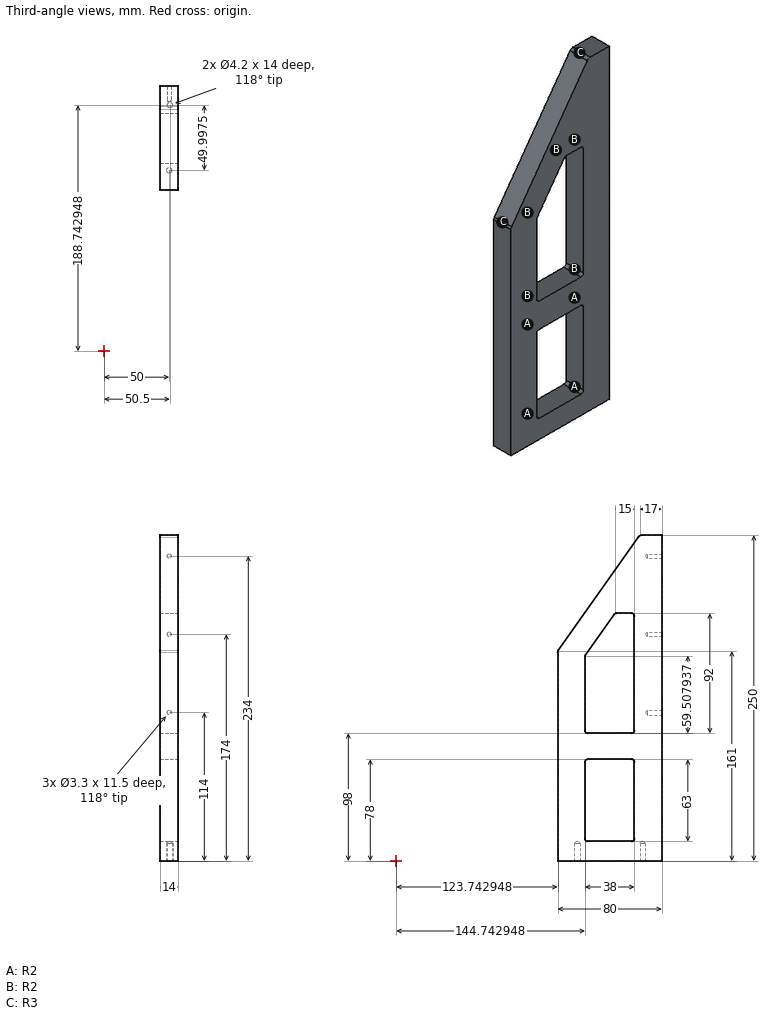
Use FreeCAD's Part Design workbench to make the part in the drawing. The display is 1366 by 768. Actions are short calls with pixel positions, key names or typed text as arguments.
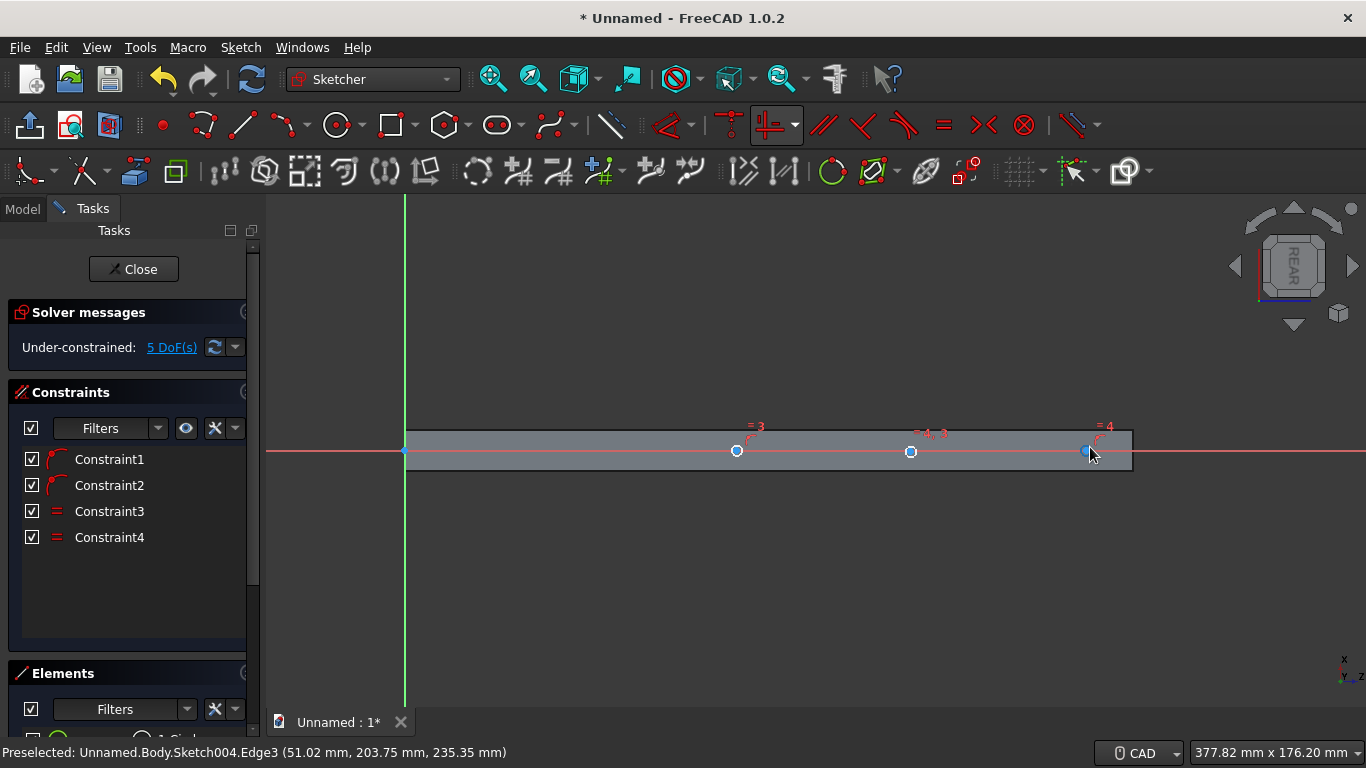
click(911, 452)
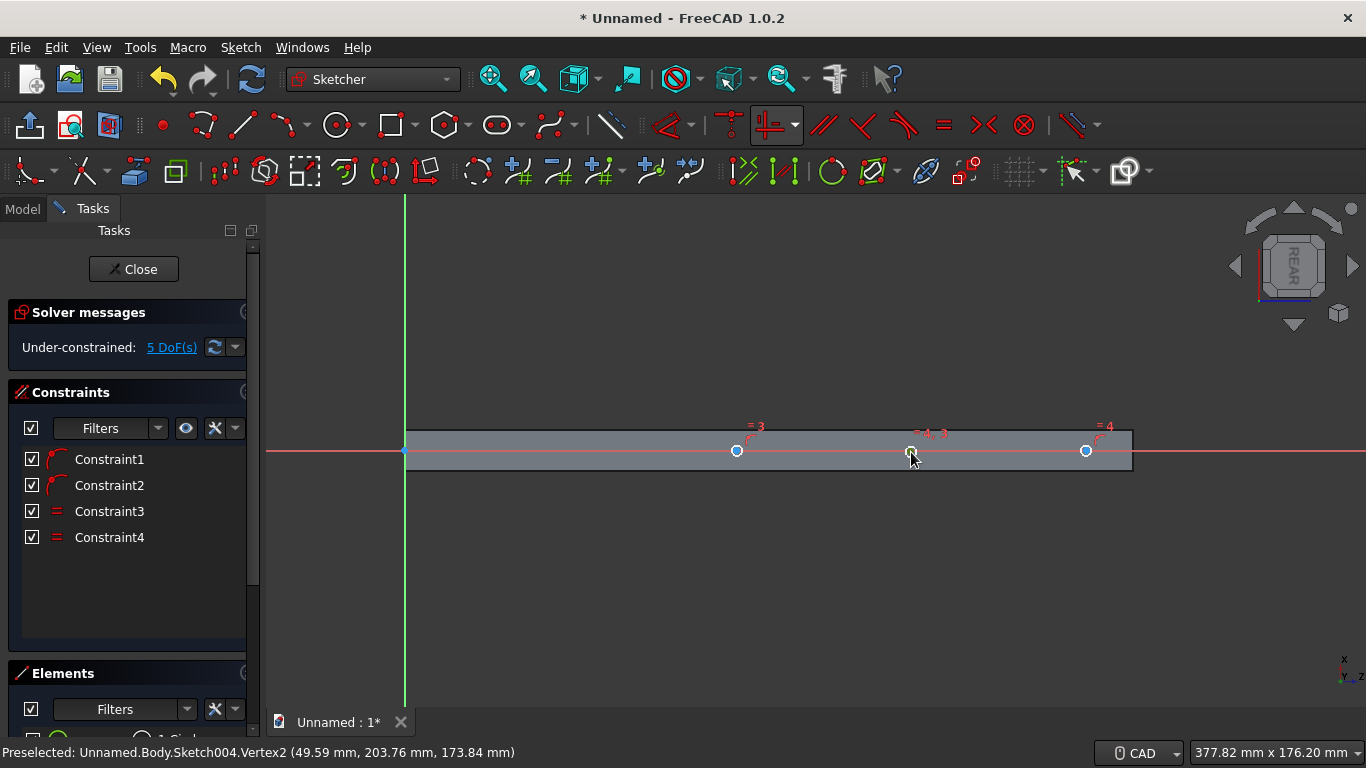
click(359, 451)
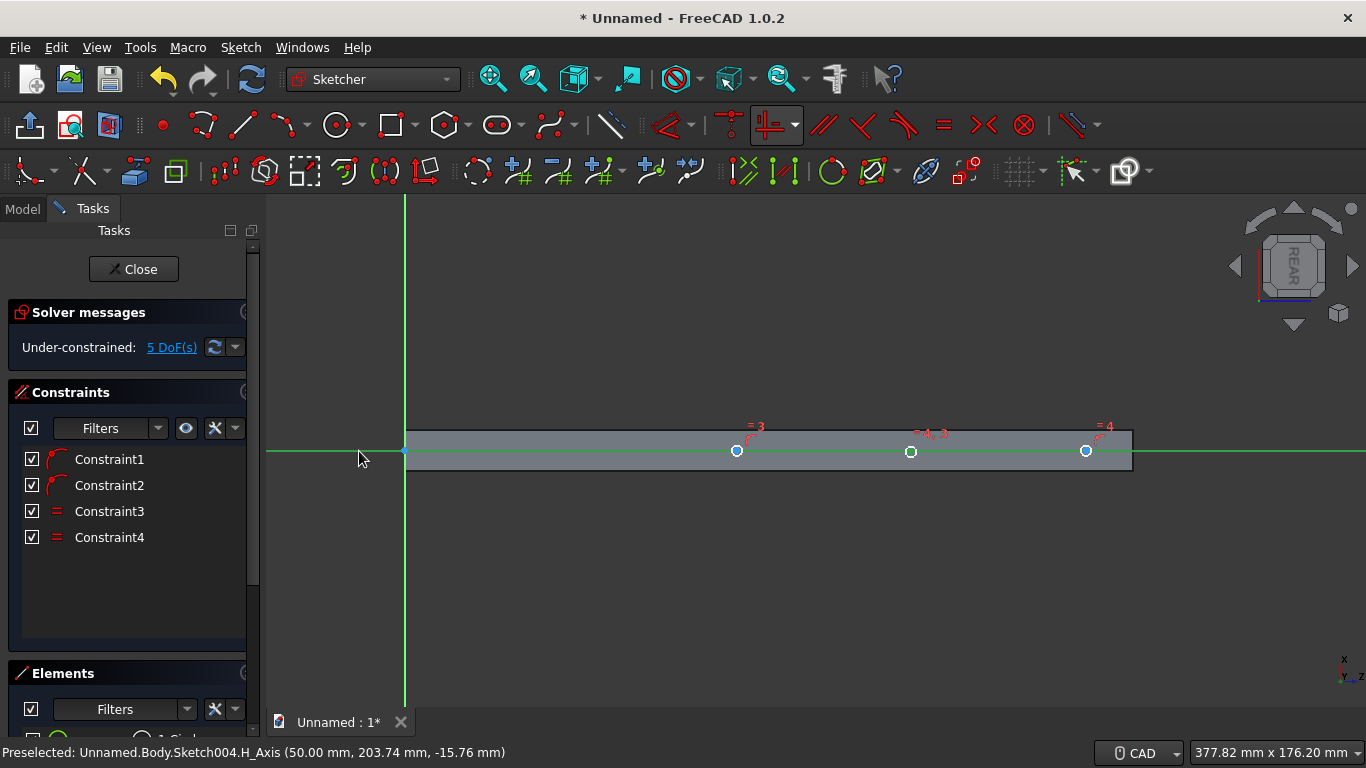
click(730, 126)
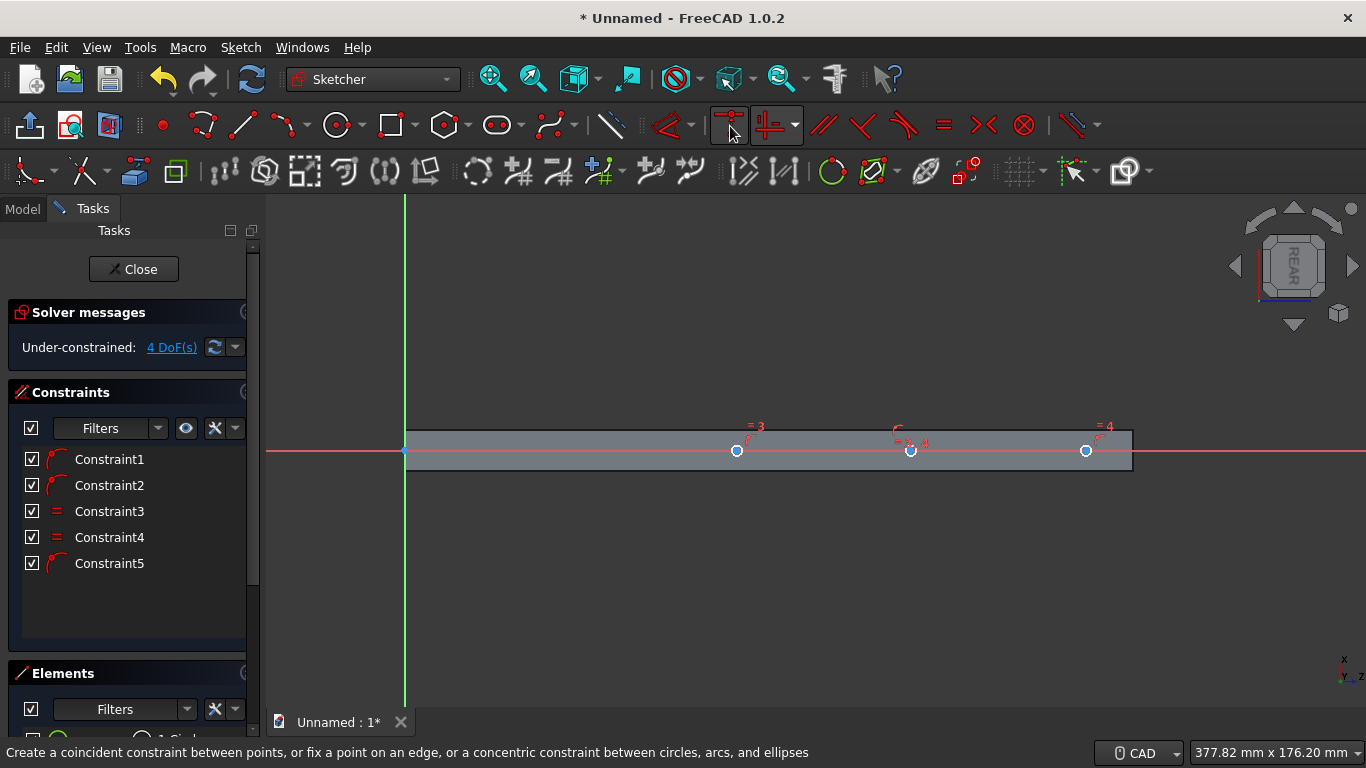
click(666, 126)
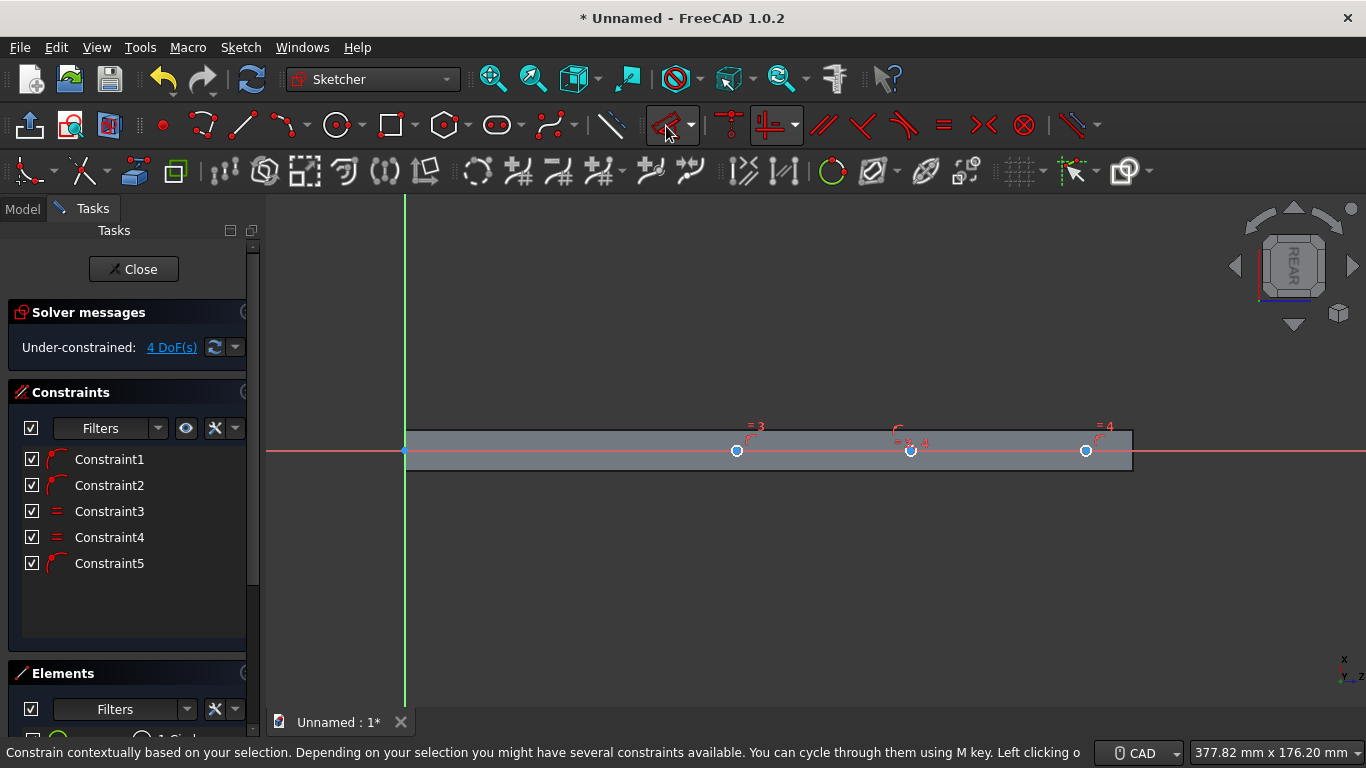
scroll(741, 454, up, 8)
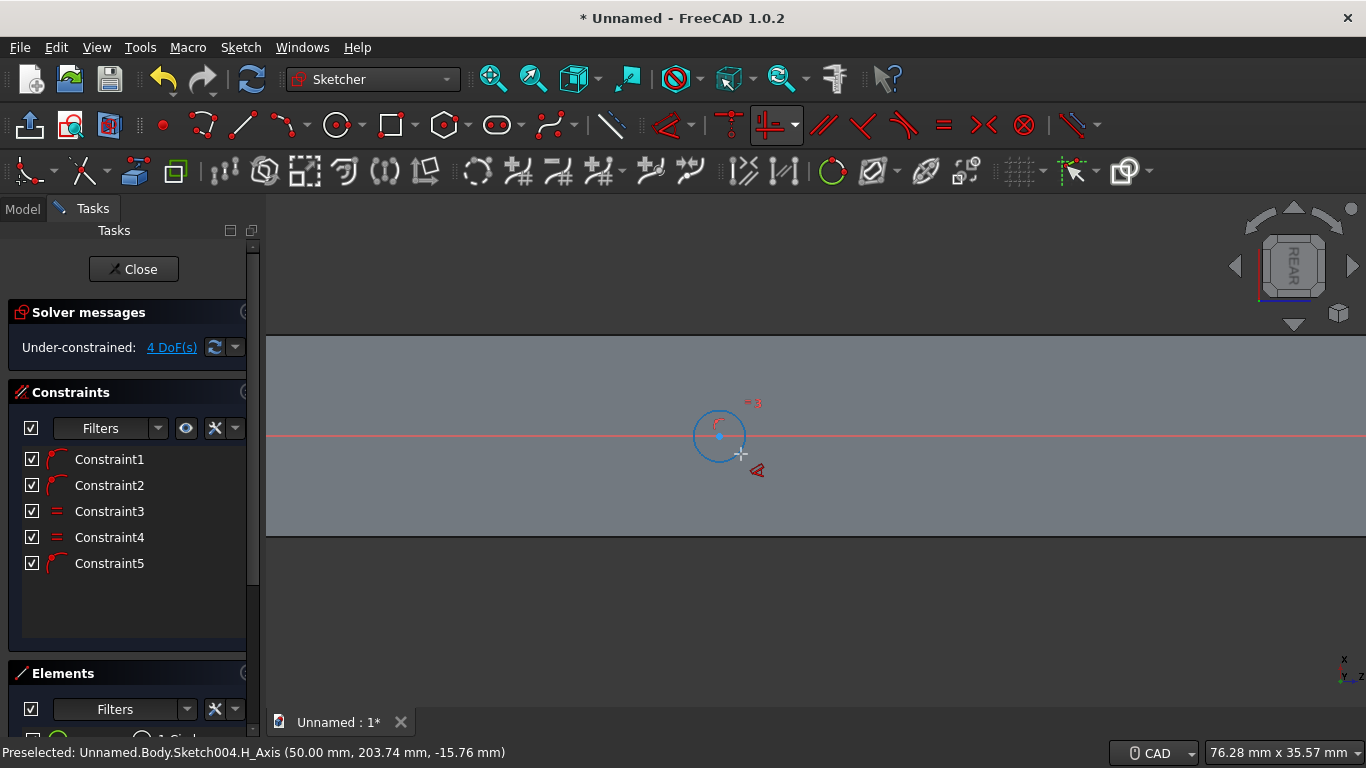
click(738, 454)
click(761, 476)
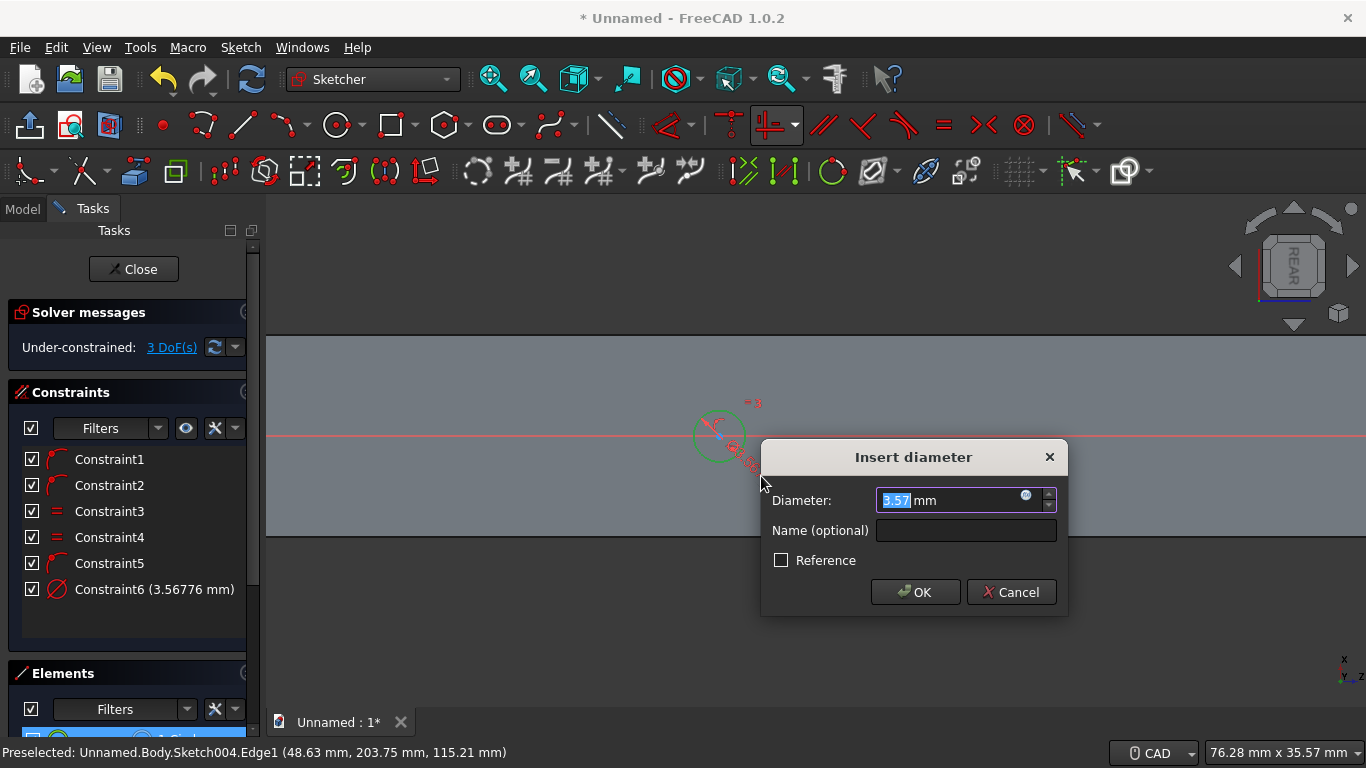
text(3.3)
key(Return)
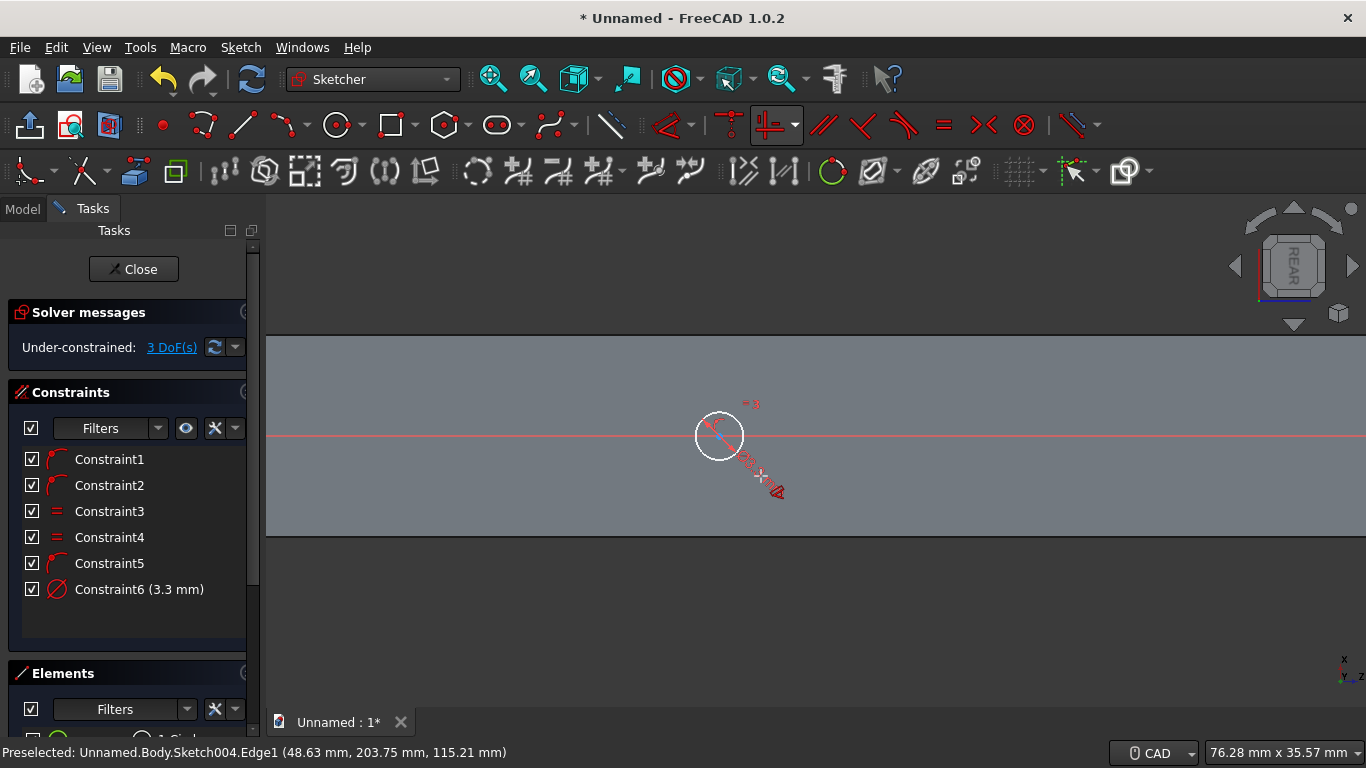
scroll(741, 454, down, 8)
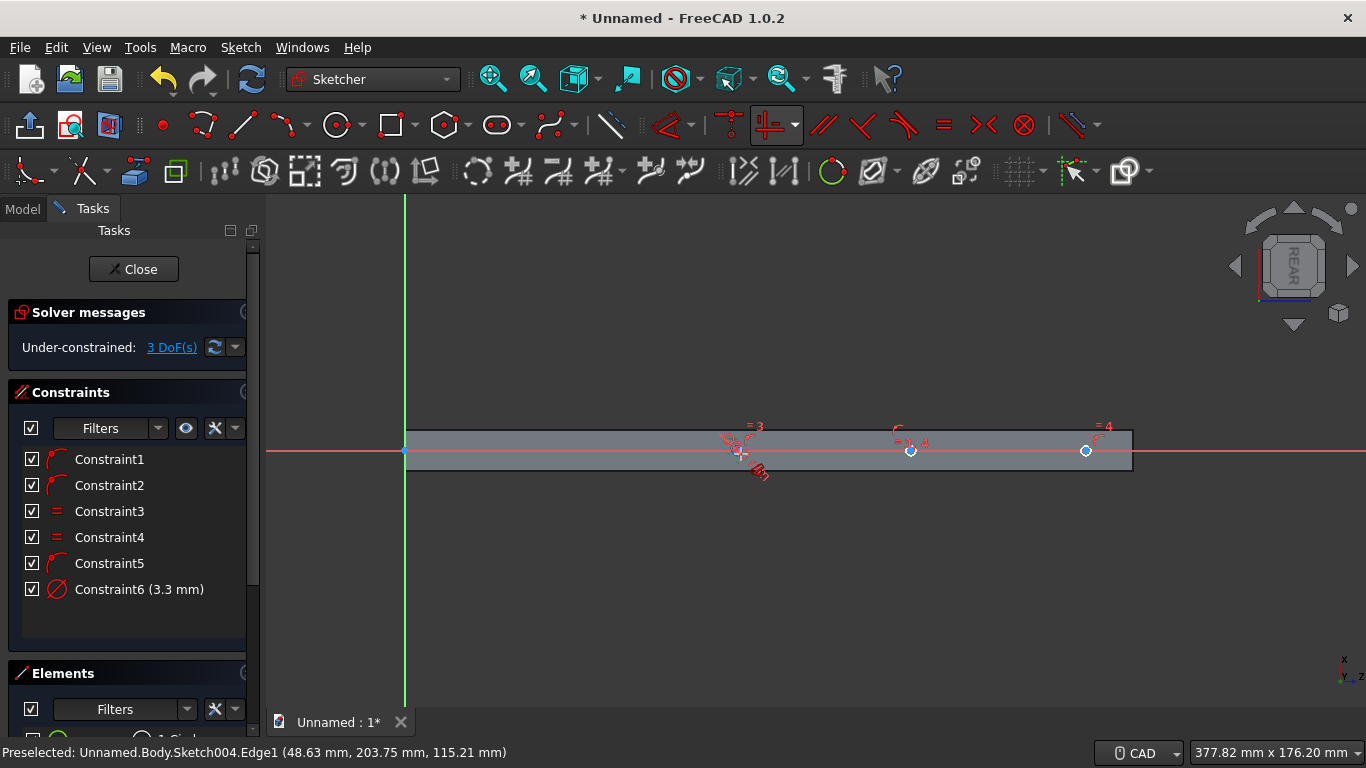
click(737, 451)
click(571, 485)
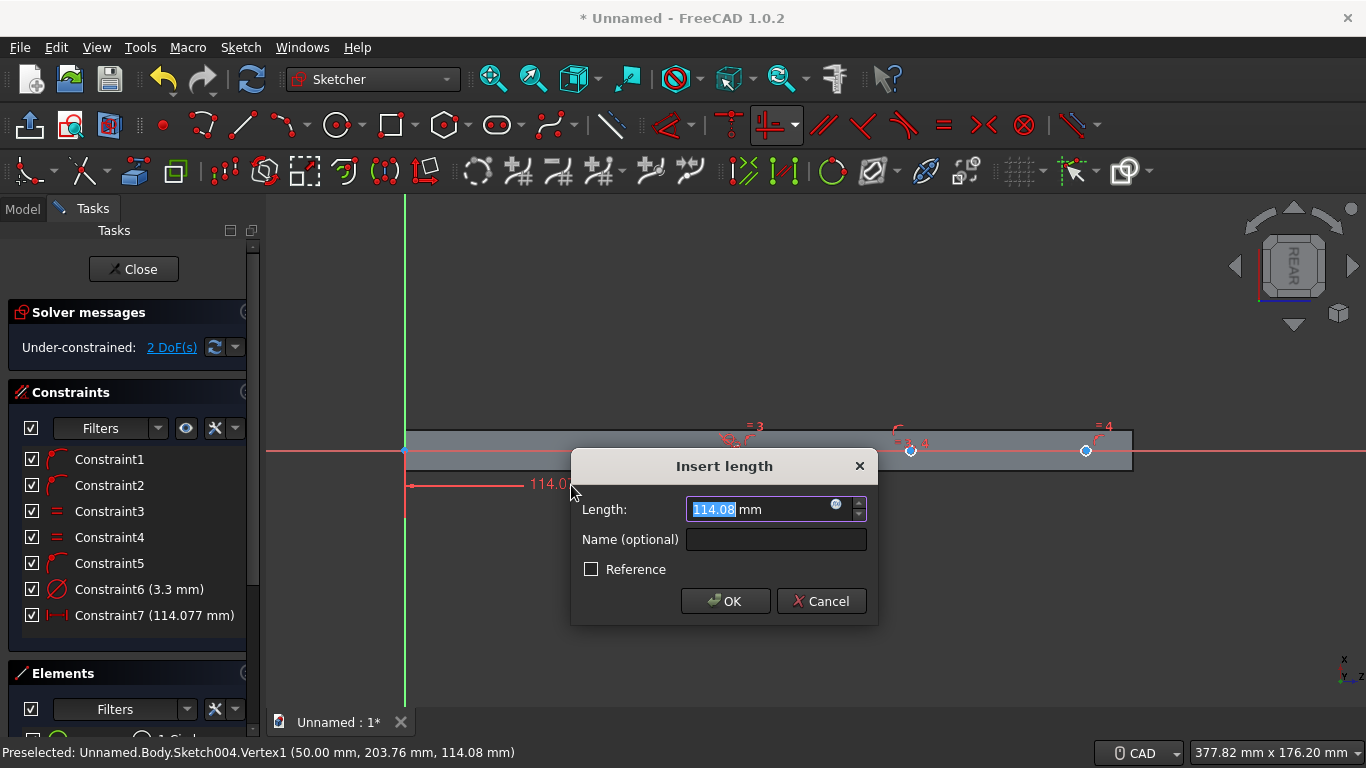
text(114)
key(Return)